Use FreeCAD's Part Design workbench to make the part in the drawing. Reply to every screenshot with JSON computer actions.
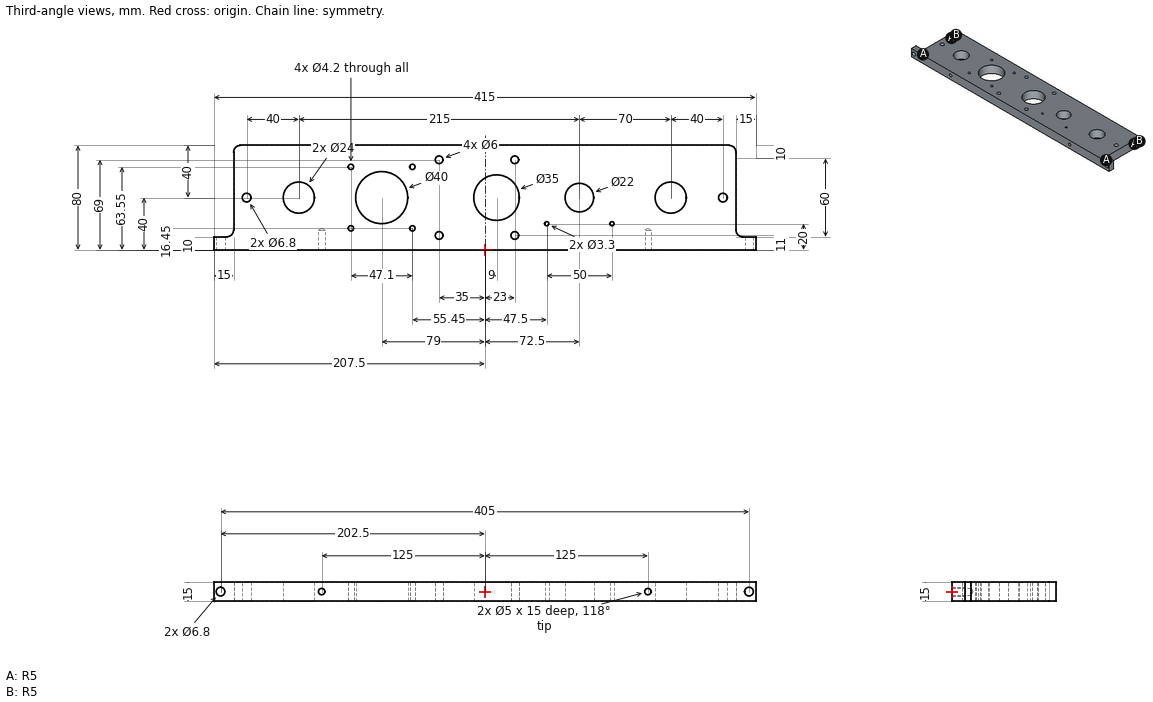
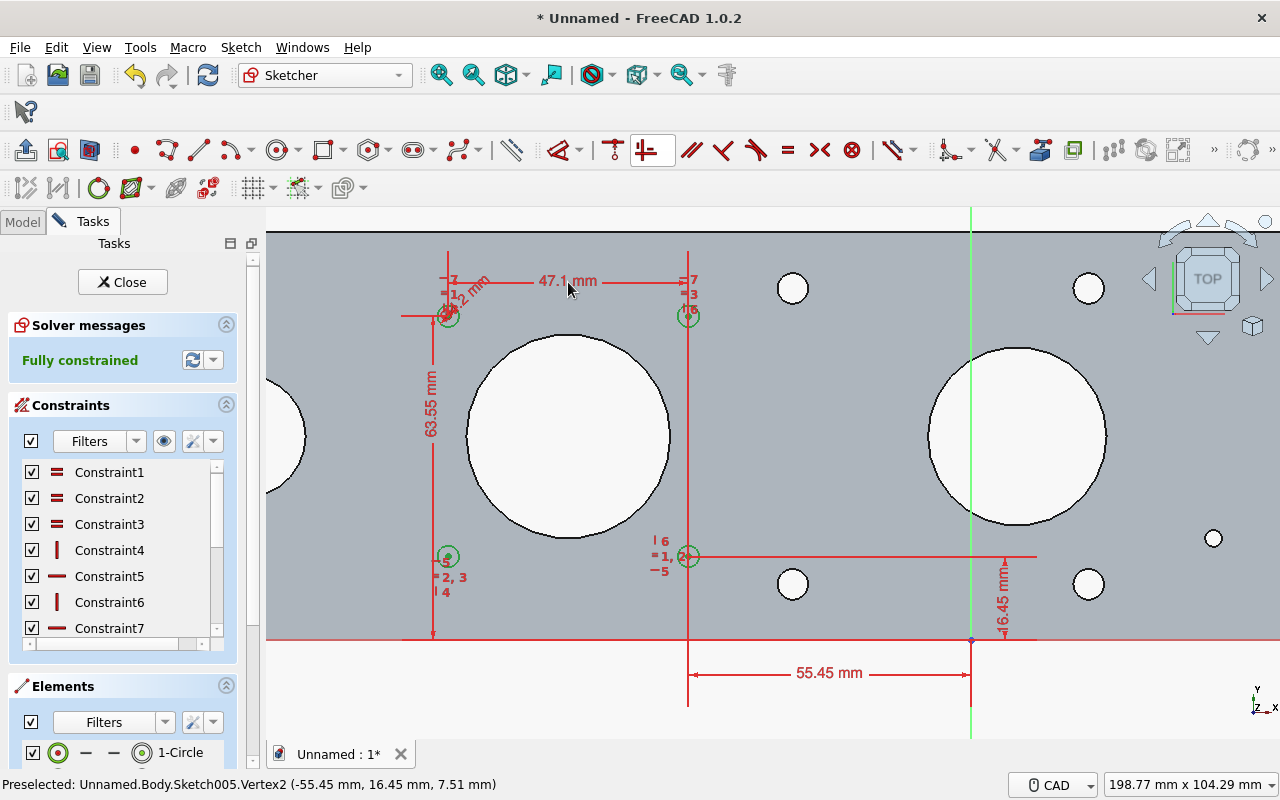
{"action": "left_click", "coordinate": [123, 282]}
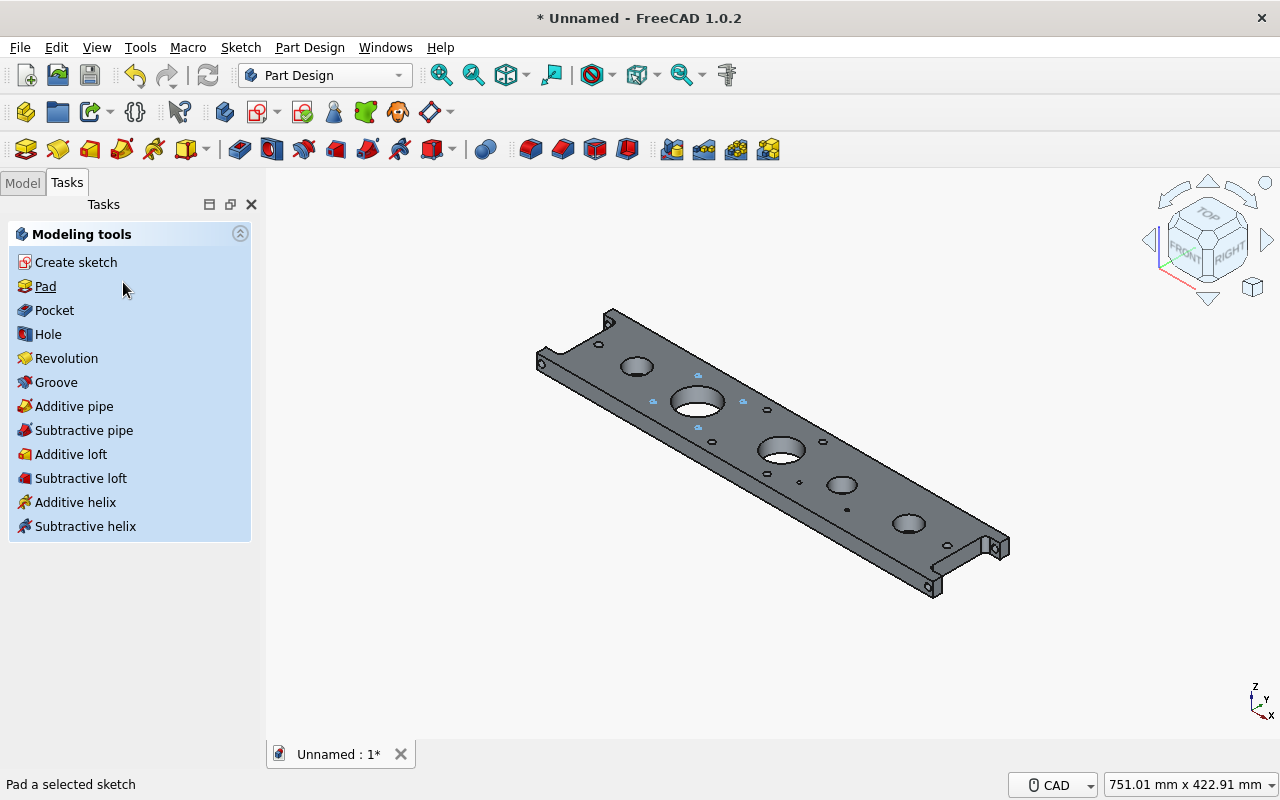
{"action": "left_click", "coordinate": [272, 150]}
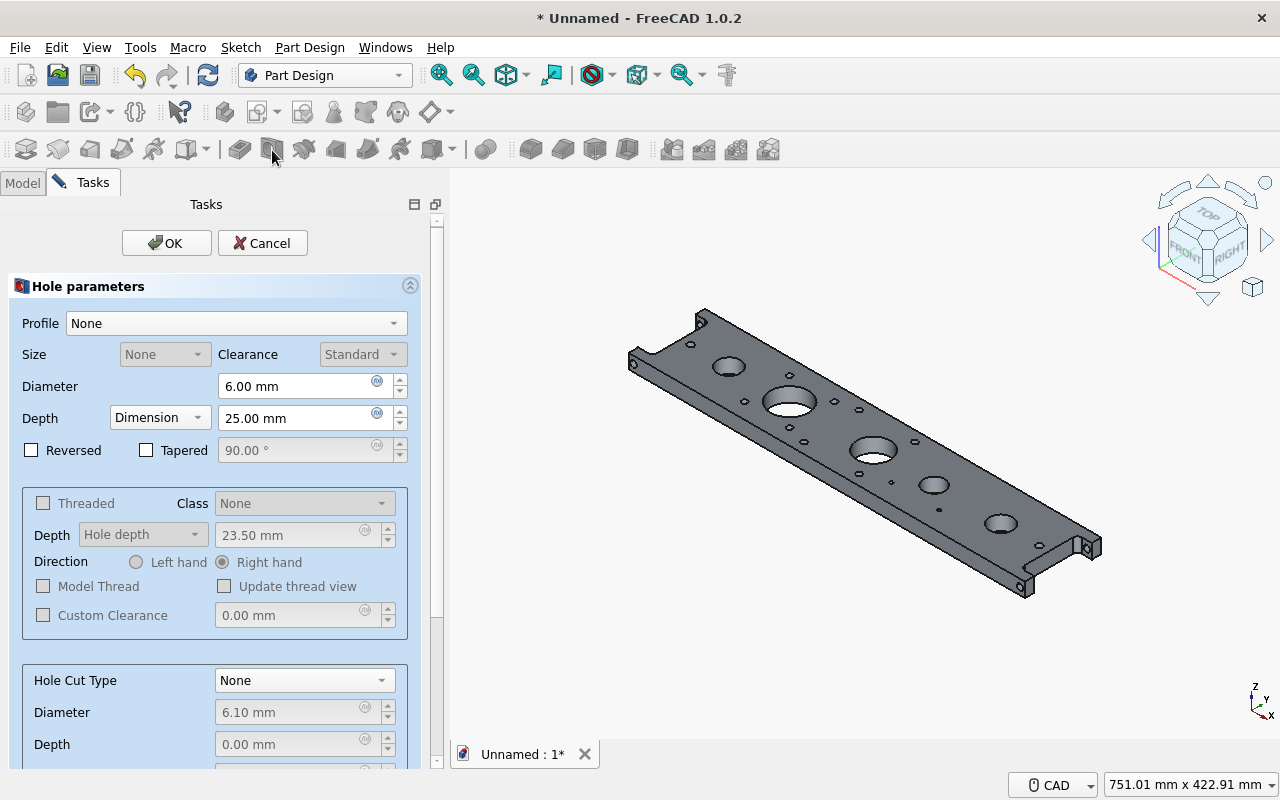
{"action": "triple_click", "coordinate": [305, 386]}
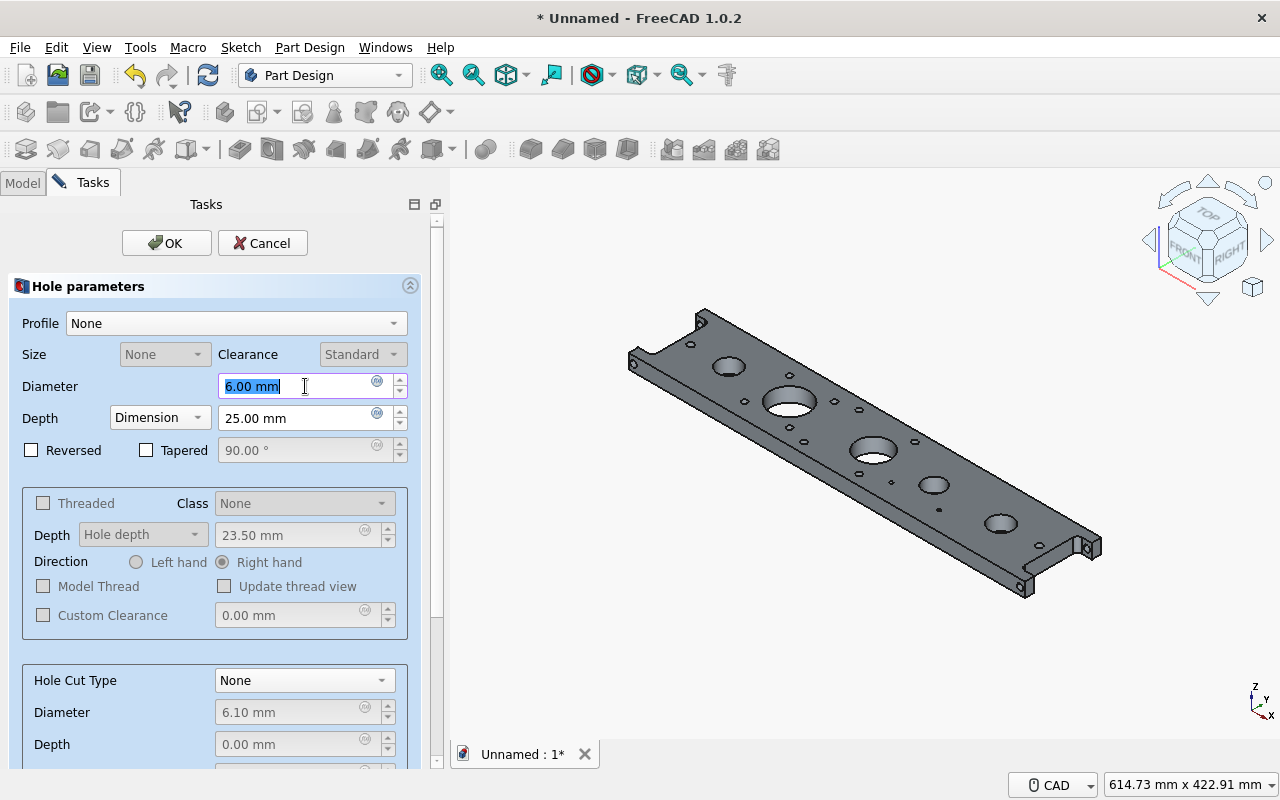
{"action": "type", "text": "4.2"}
{"action": "key", "text": "Tab"}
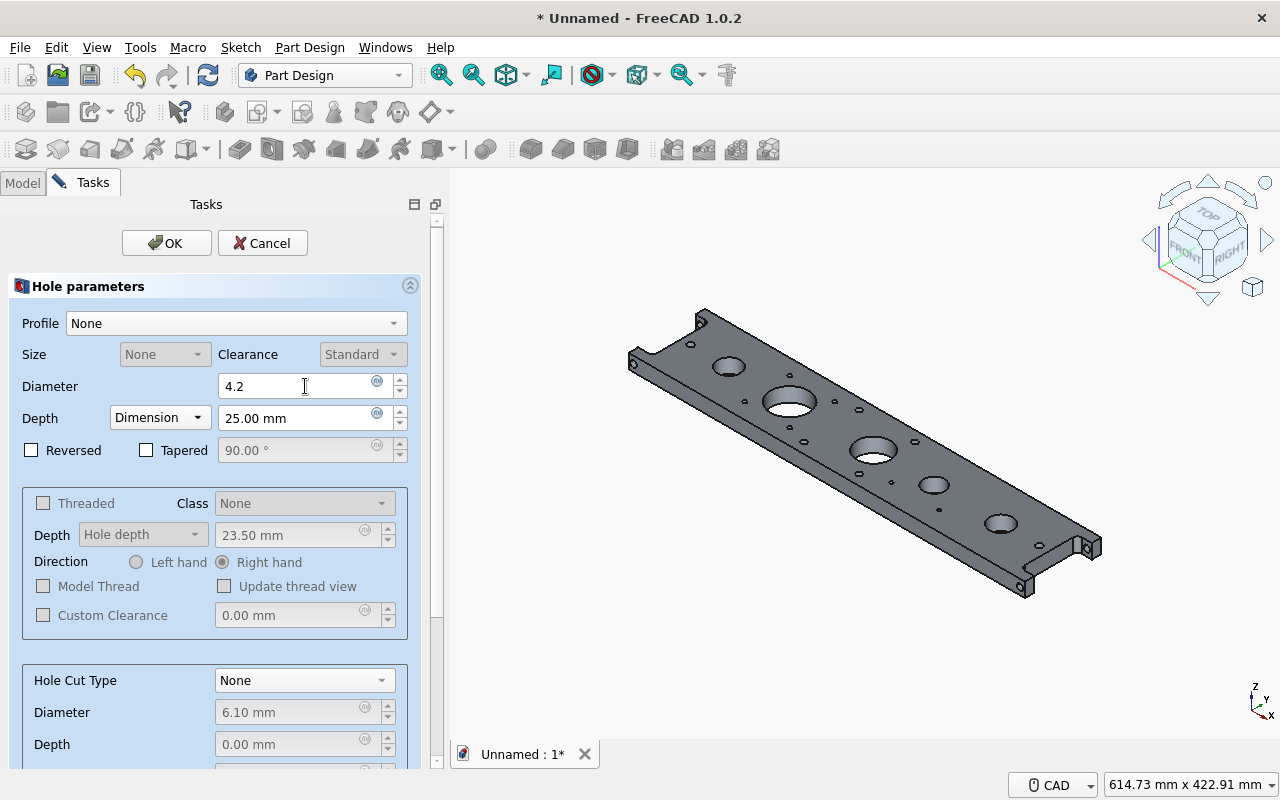
{"action": "left_click", "coordinate": [161, 418]}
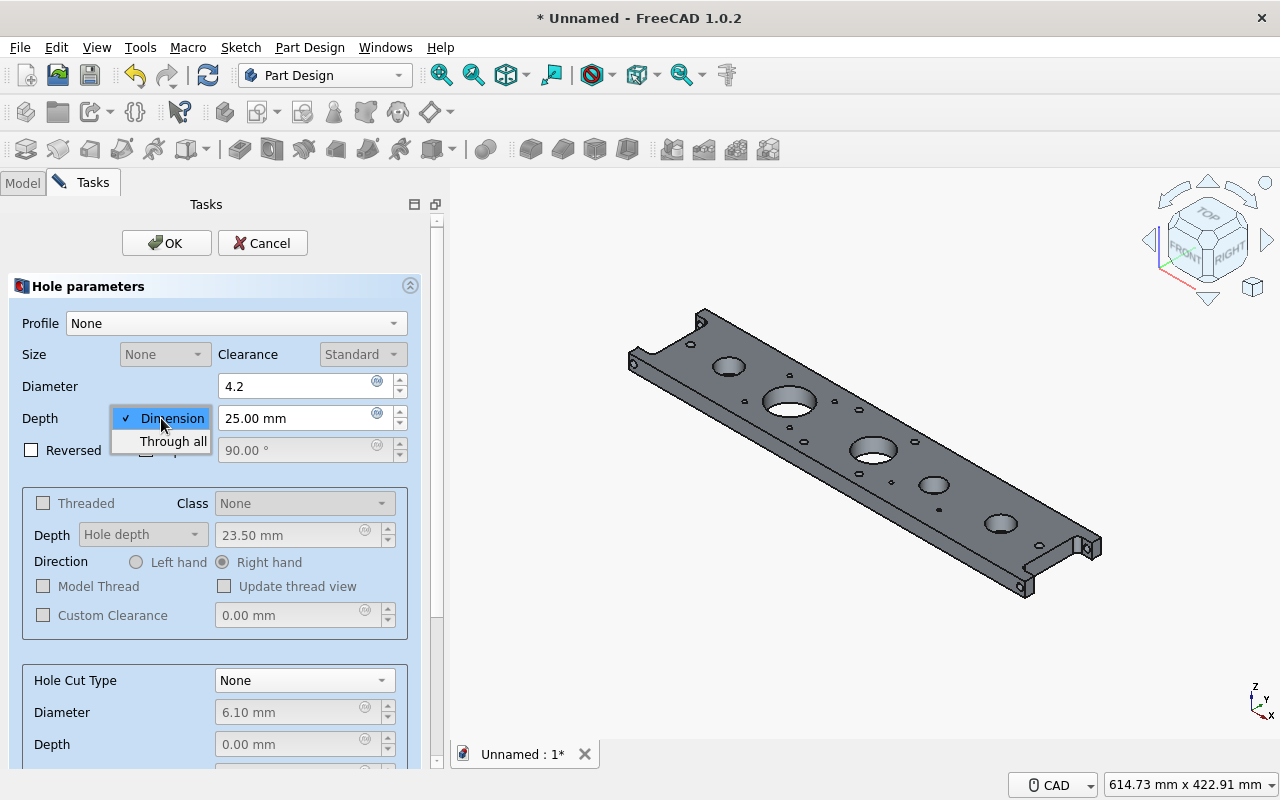
{"action": "left_click", "coordinate": [160, 442]}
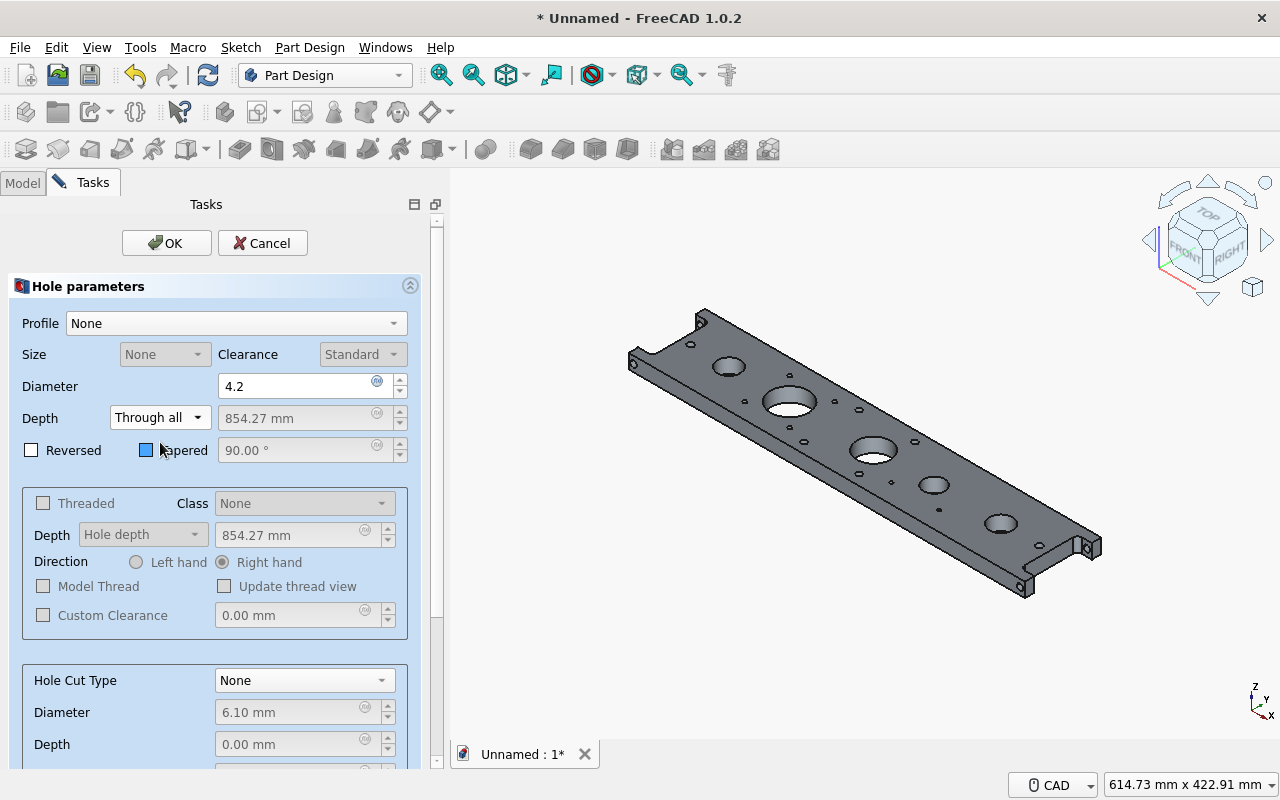
{"action": "left_click", "coordinate": [167, 243]}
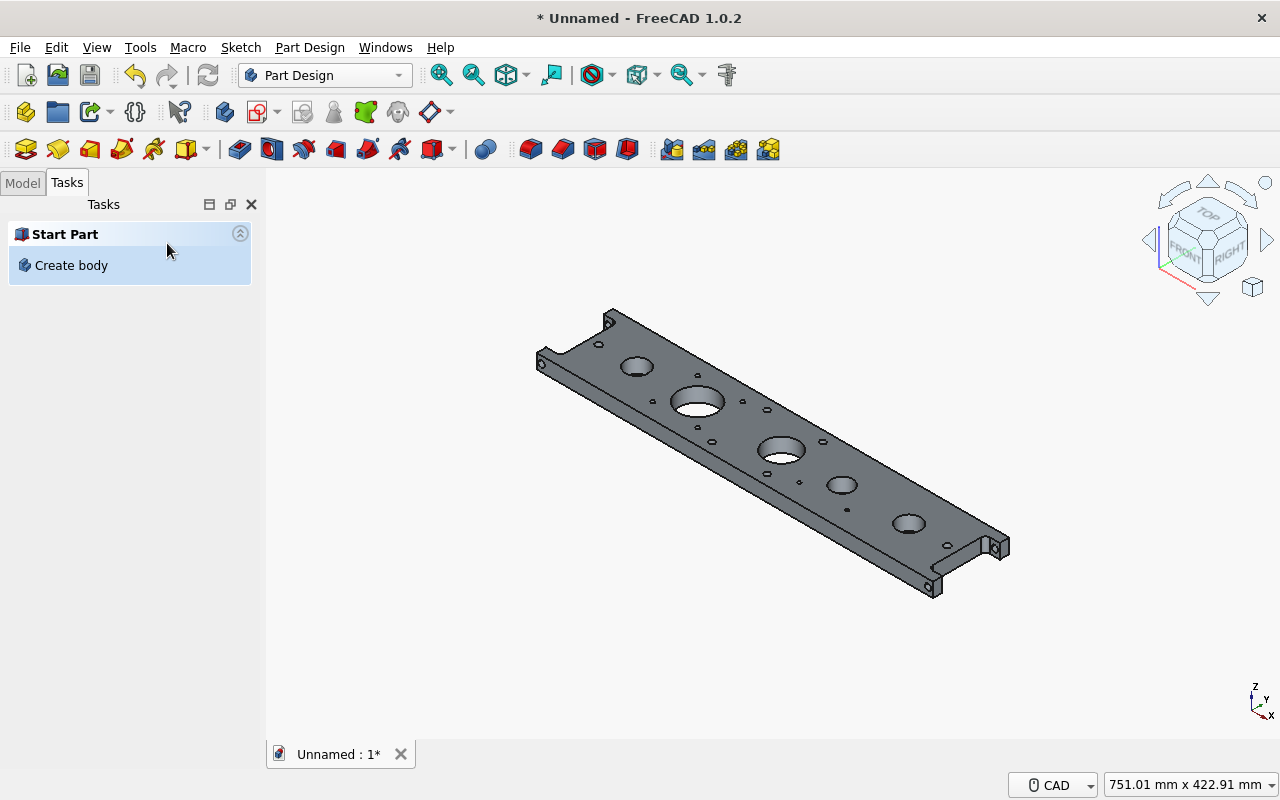
{"action": "left_click", "coordinate": [908, 497]}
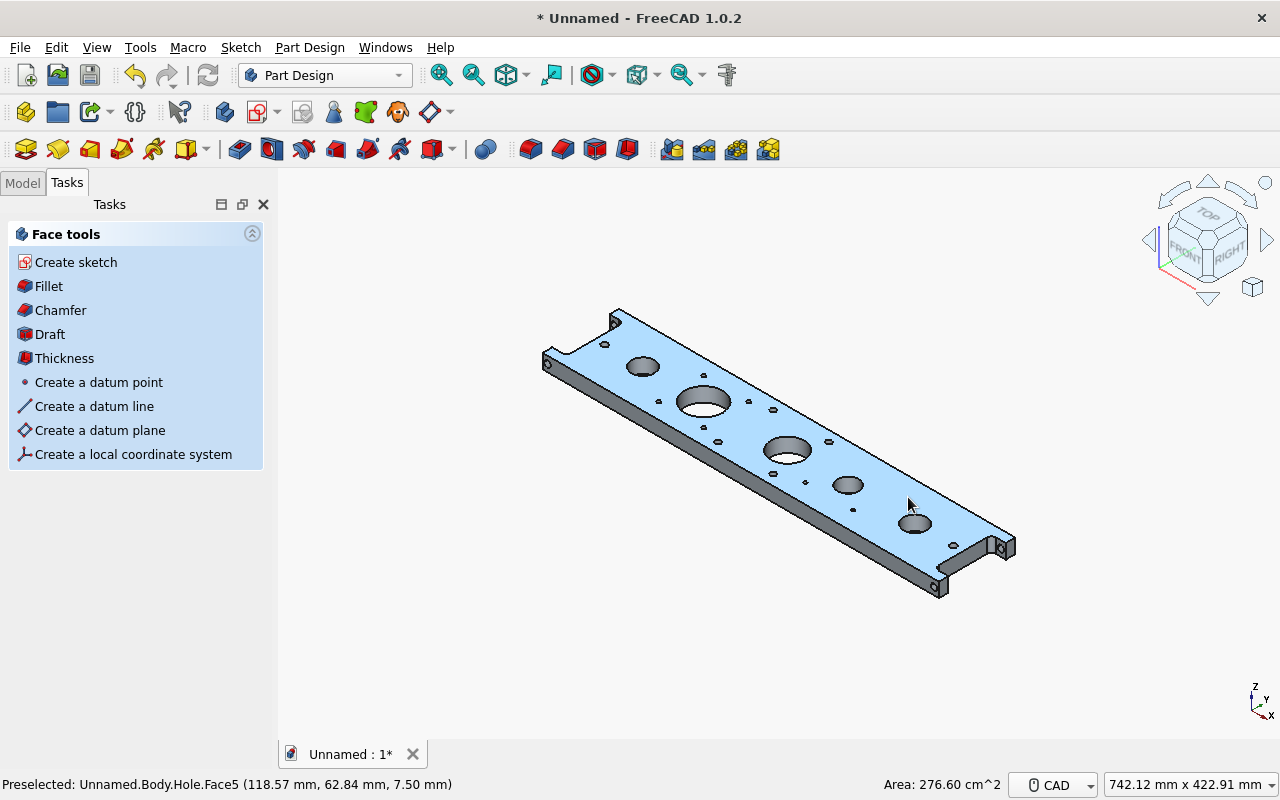
{"action": "left_click", "coordinate": [258, 112]}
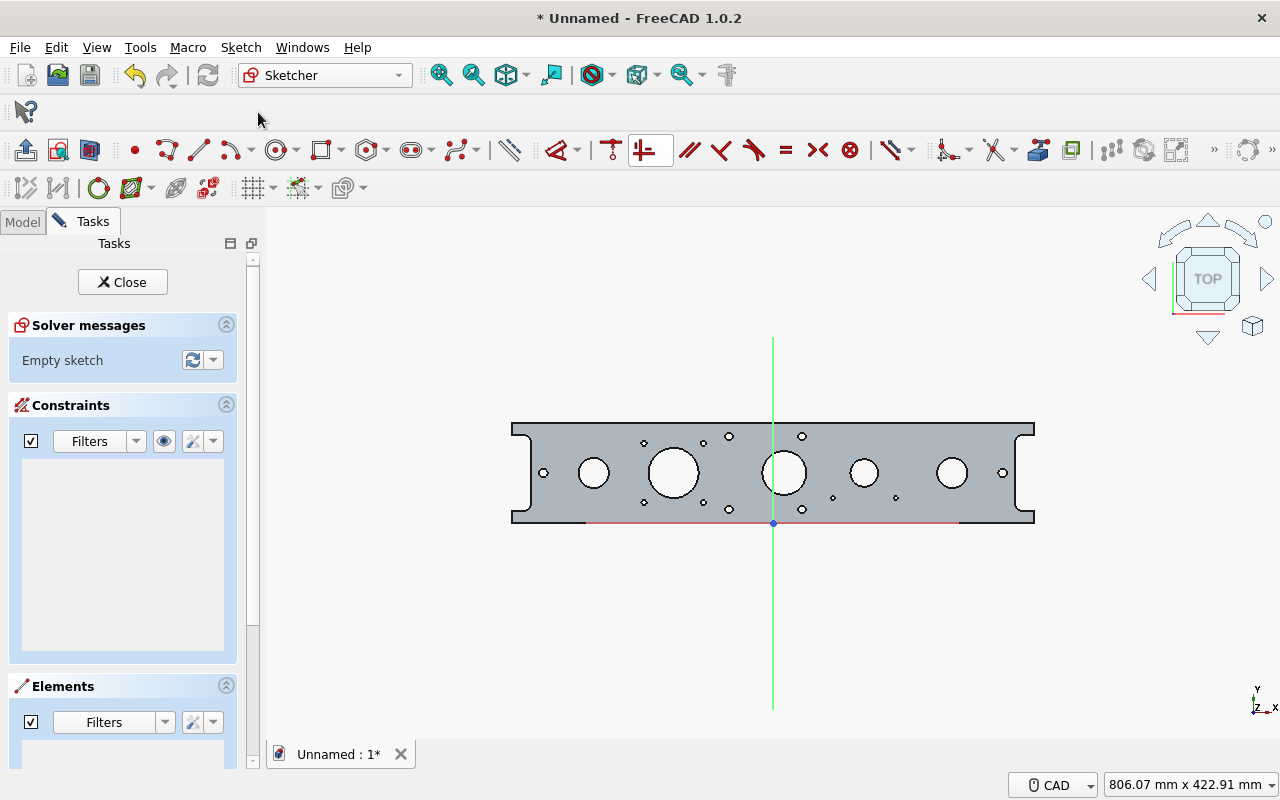
{"action": "left_click", "coordinate": [322, 150]}